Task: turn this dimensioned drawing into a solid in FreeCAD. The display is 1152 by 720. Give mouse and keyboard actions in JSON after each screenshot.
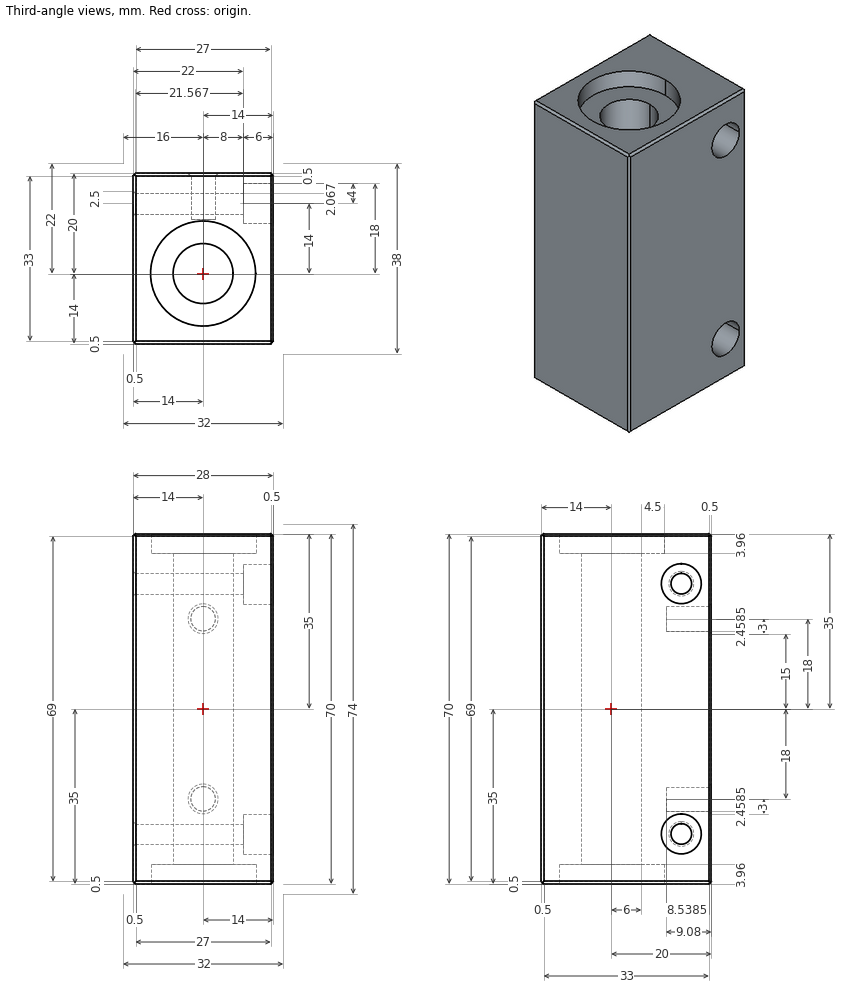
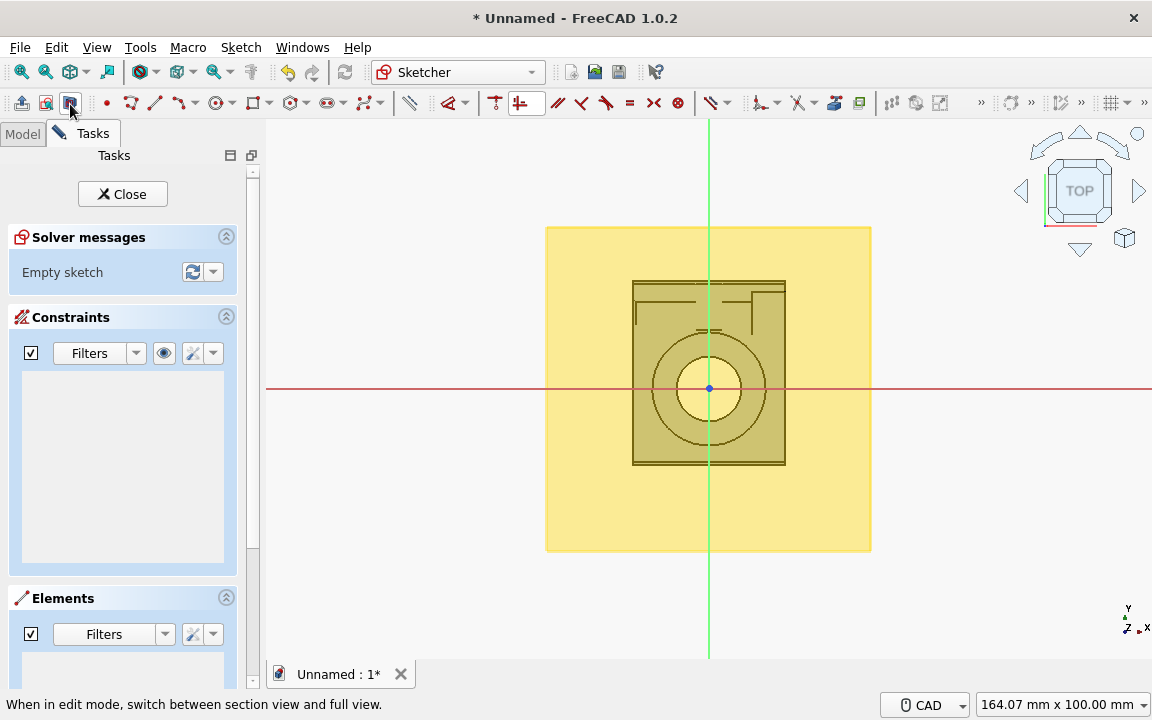
{"action": "scroll", "coordinate": [686, 319], "scroll_direction": "up", "scroll_amount": 5}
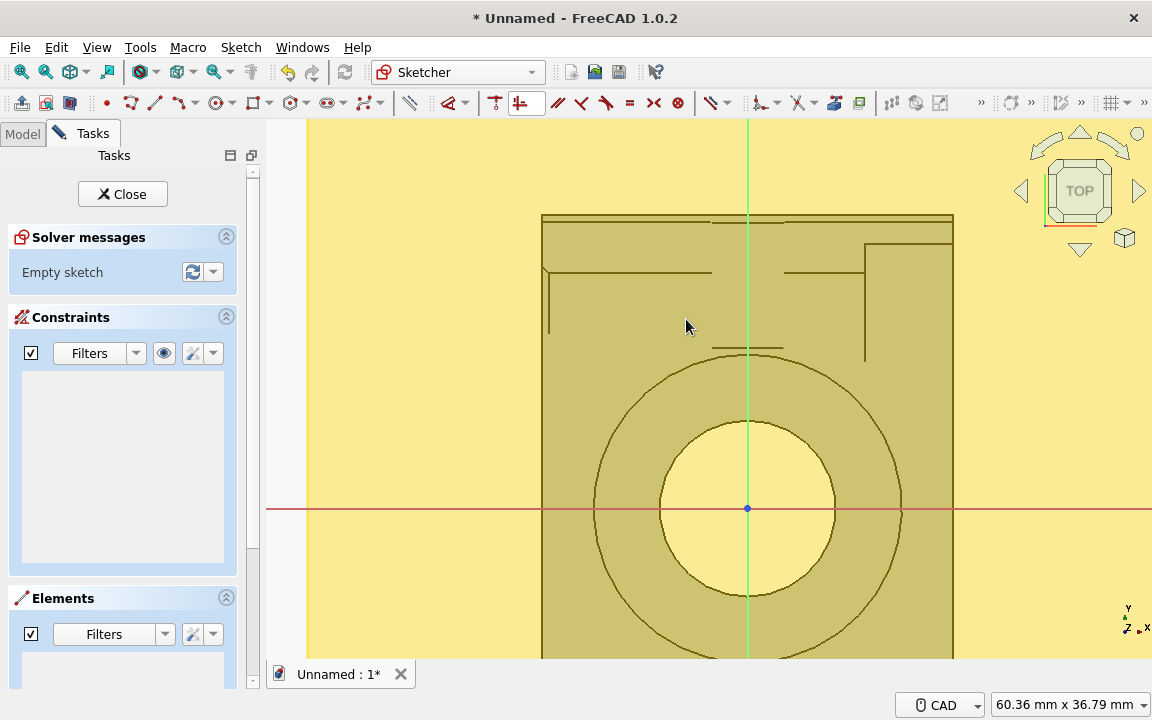
{"action": "left_click", "coordinate": [132, 104]}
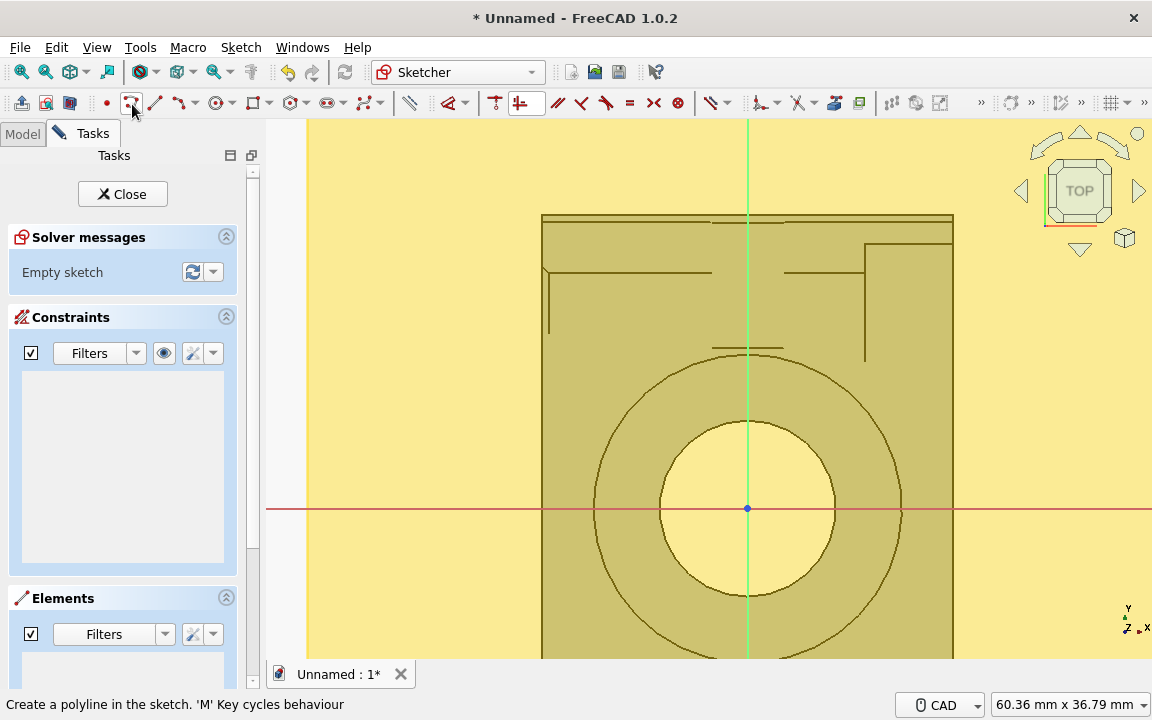
{"action": "left_click", "coordinate": [865, 303]}
{"action": "left_click", "coordinate": [865, 273]}
{"action": "left_click", "coordinate": [549, 273]}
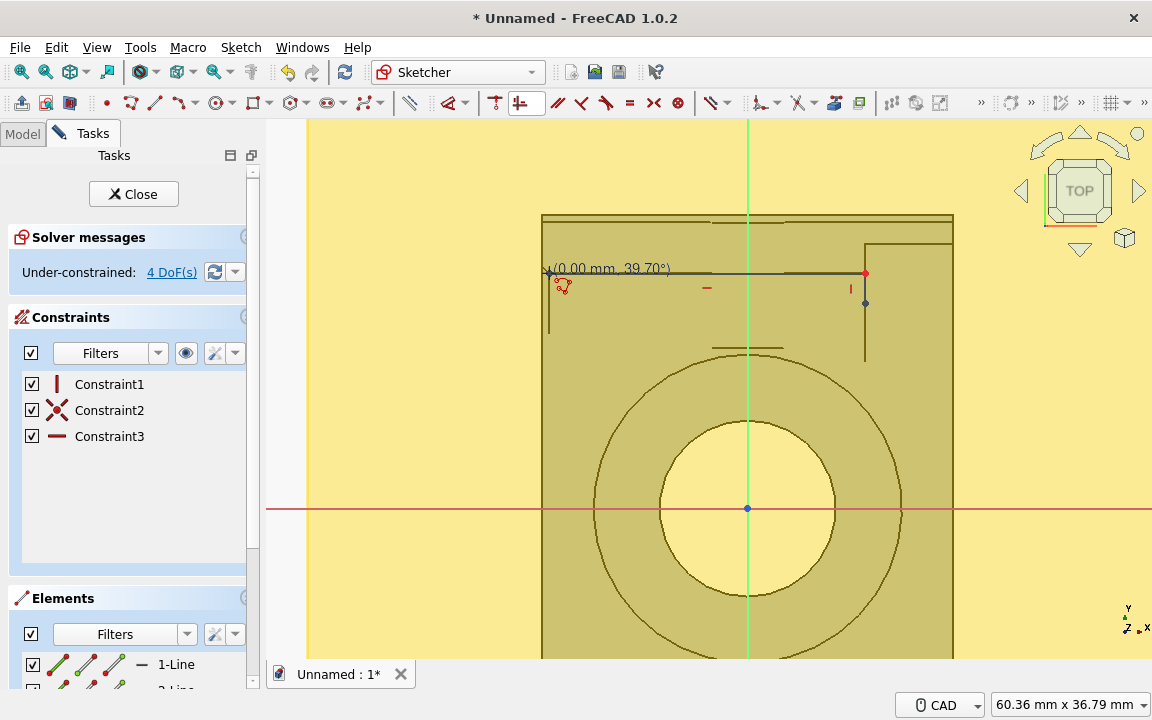
{"action": "scroll", "coordinate": [542, 266], "scroll_direction": "up", "scroll_amount": 3}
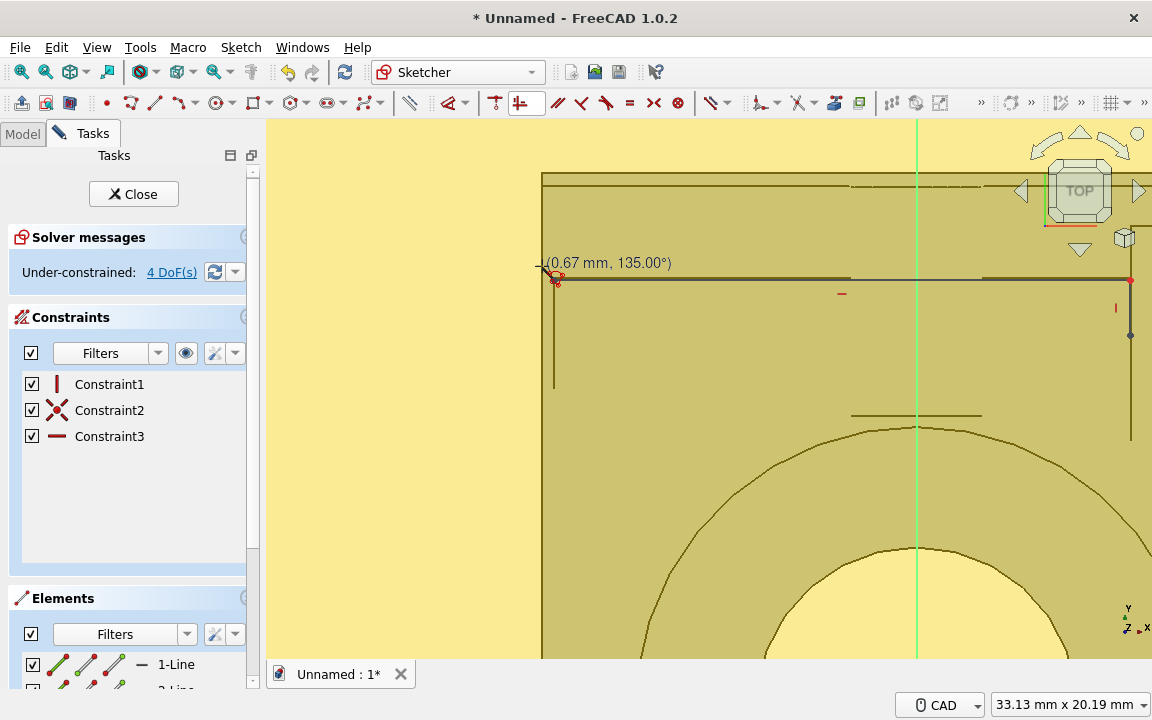
{"action": "left_click", "coordinate": [542, 267]}
{"action": "left_click", "coordinate": [542, 333]}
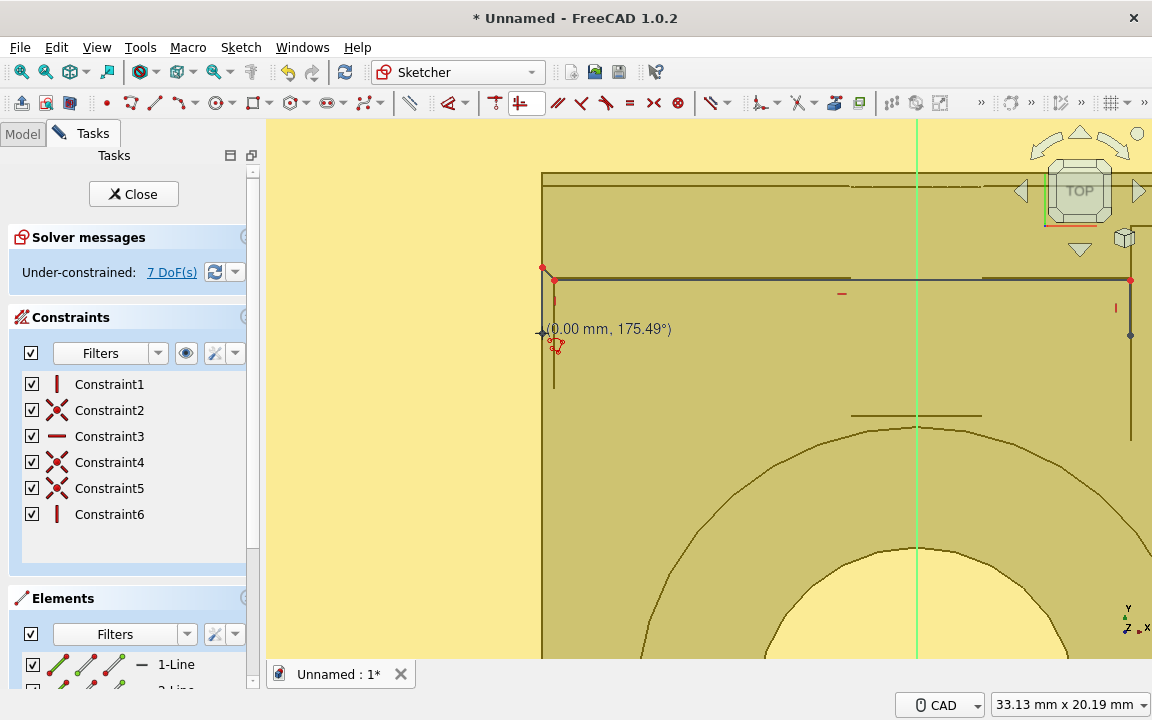
{"action": "scroll", "coordinate": [545, 270], "scroll_direction": "down", "scroll_amount": 3}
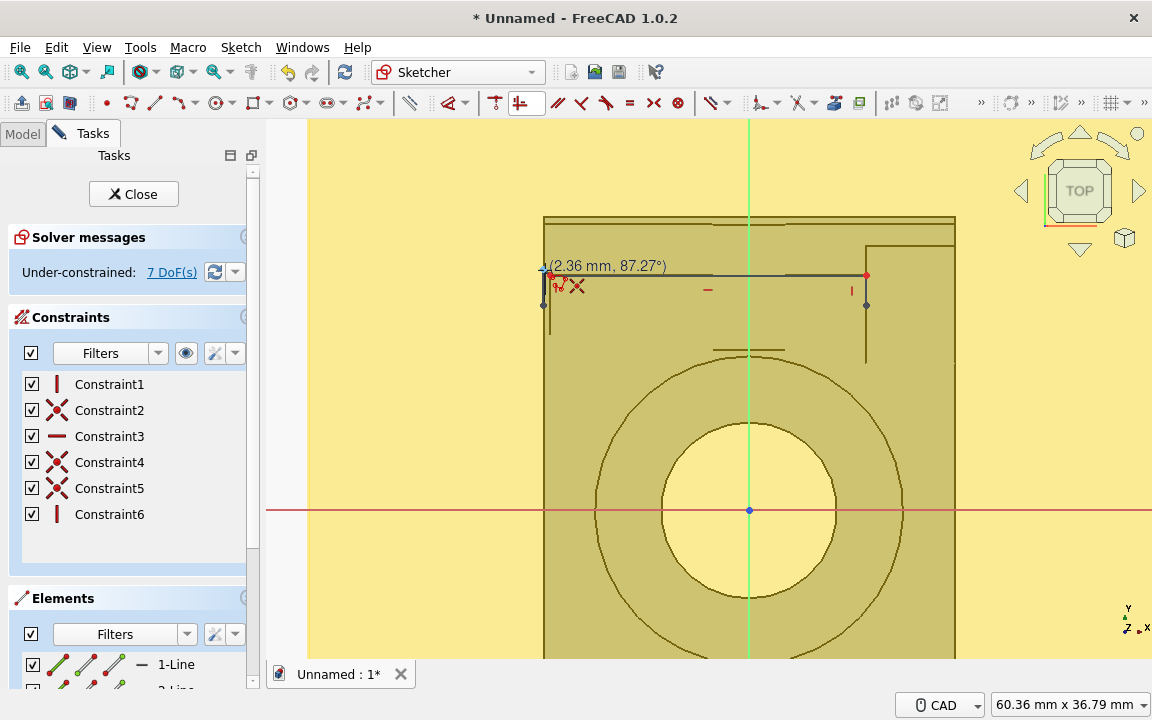
{"action": "left_click", "coordinate": [866, 306]}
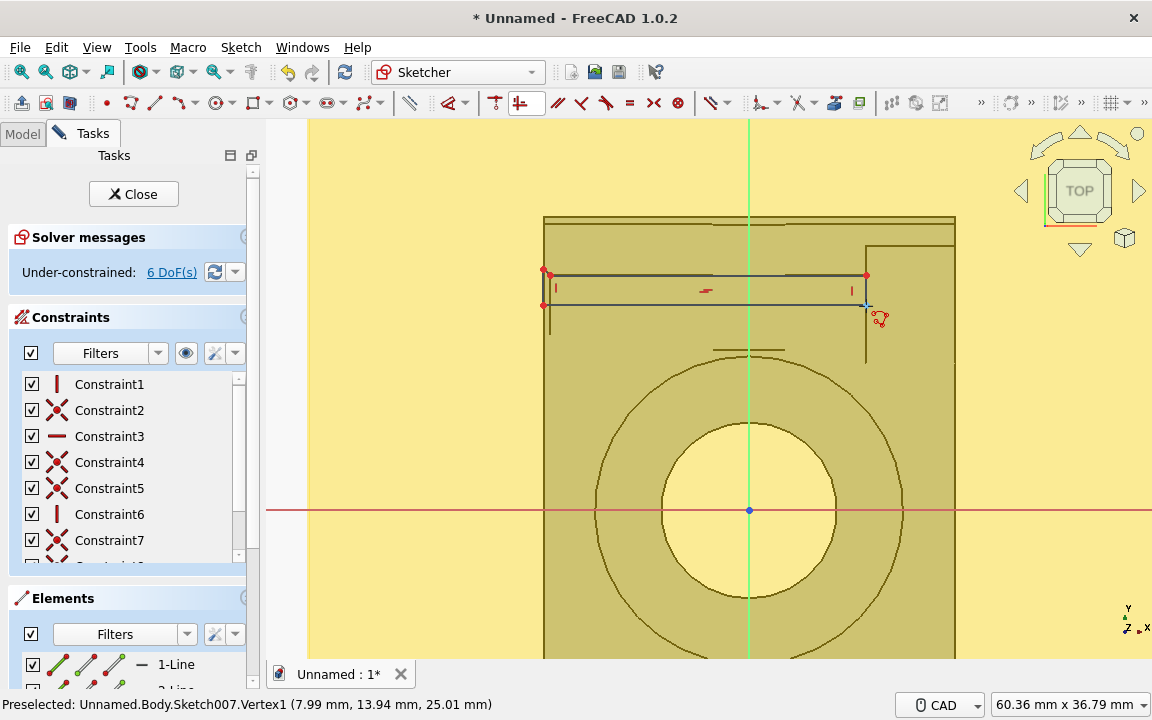
{"action": "left_click", "coordinate": [156, 104]}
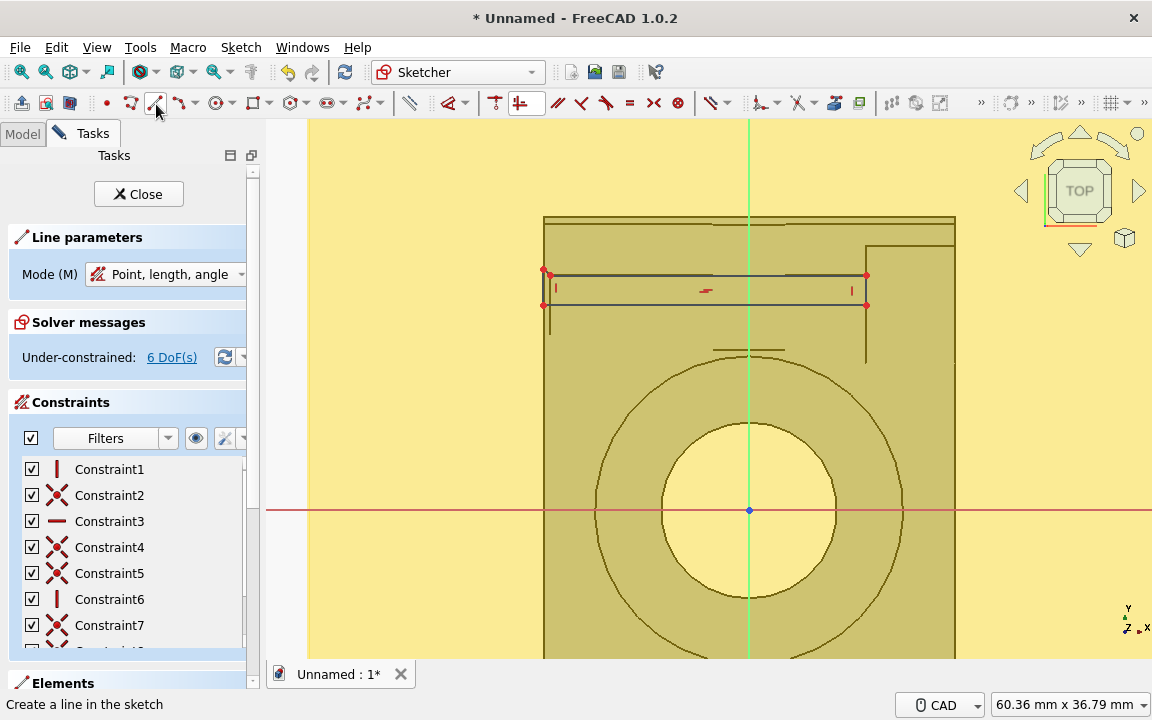
{"action": "left_click", "coordinate": [511, 305]}
{"action": "left_click", "coordinate": [414, 305]}
{"action": "key", "text": "Escape"}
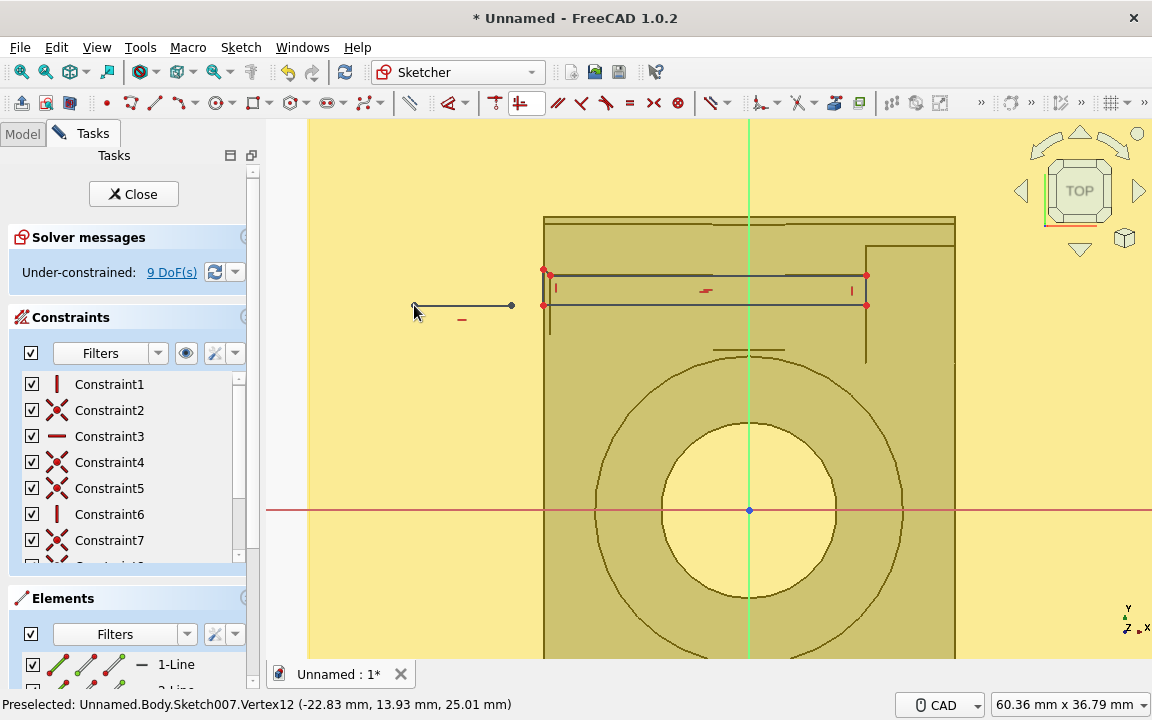
{"action": "left_click", "coordinate": [482, 306]}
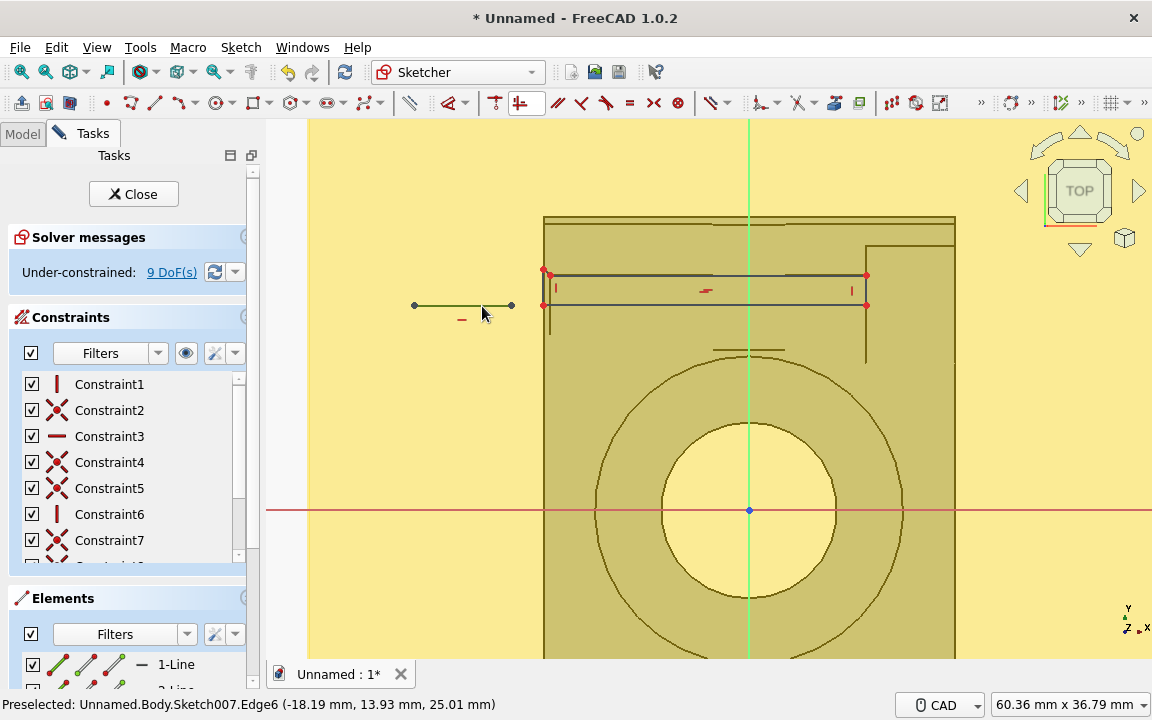
{"action": "left_click", "coordinate": [410, 104]}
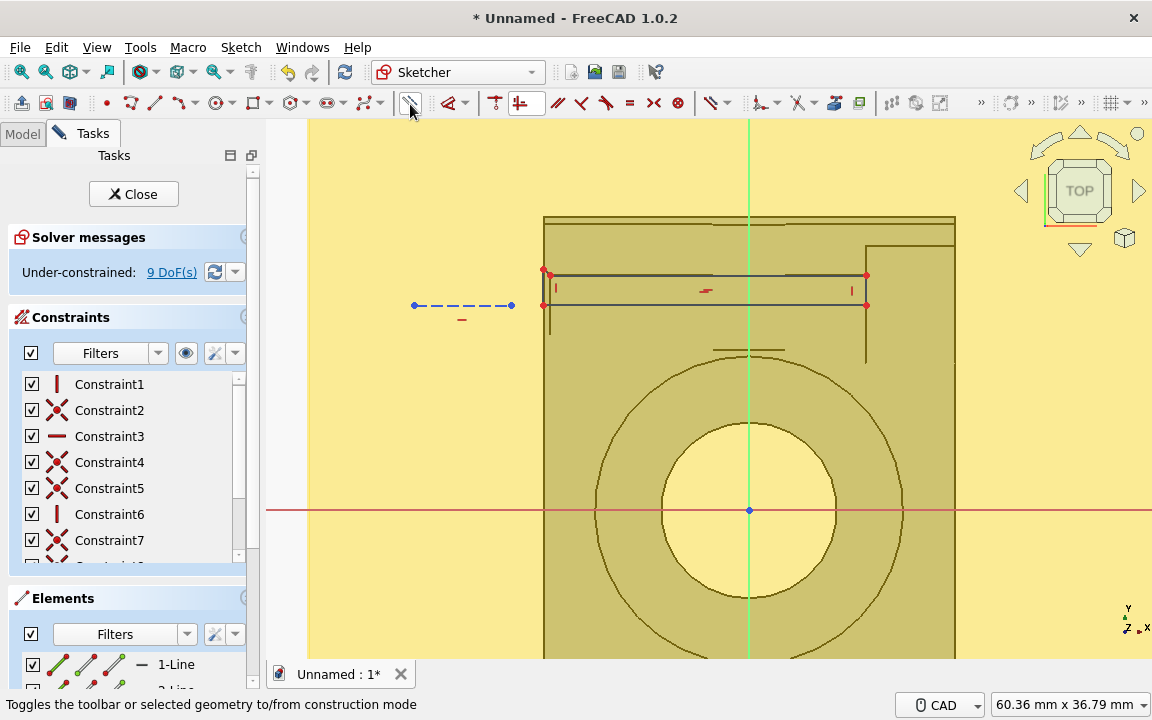
{"action": "left_click", "coordinate": [448, 104]}